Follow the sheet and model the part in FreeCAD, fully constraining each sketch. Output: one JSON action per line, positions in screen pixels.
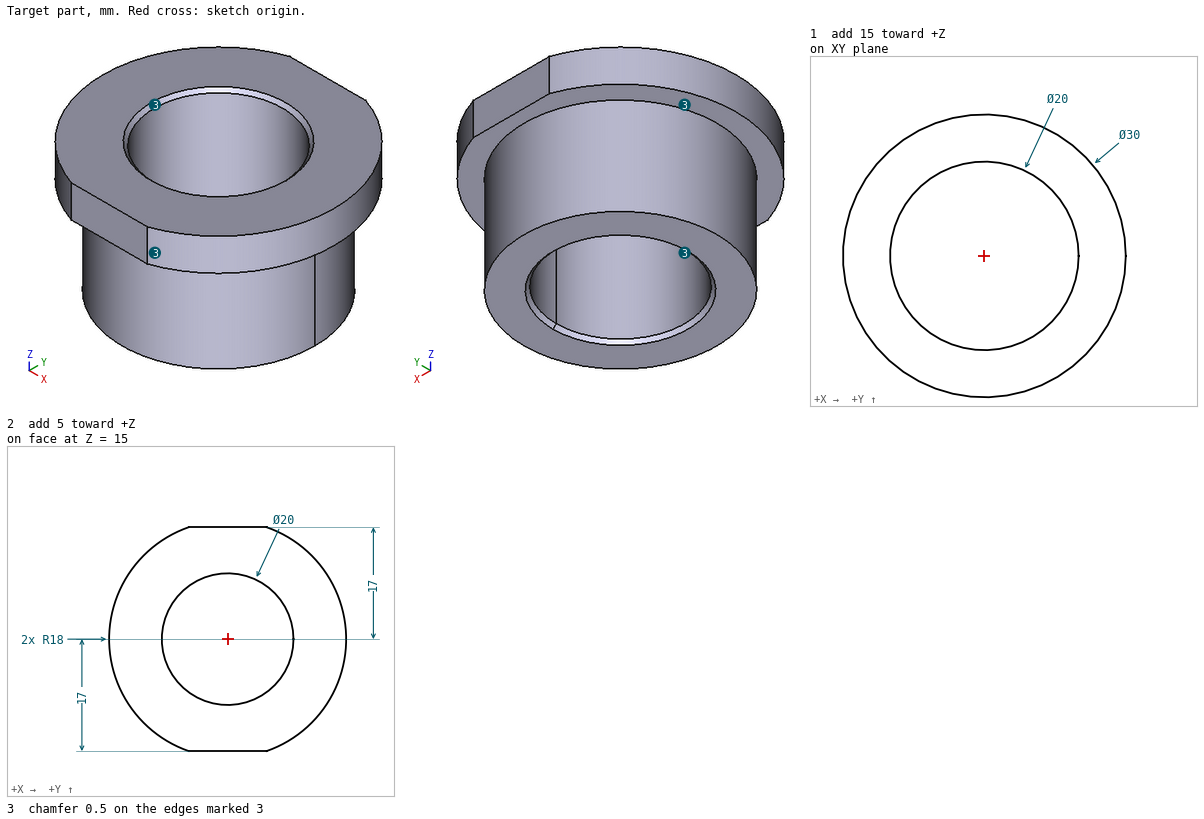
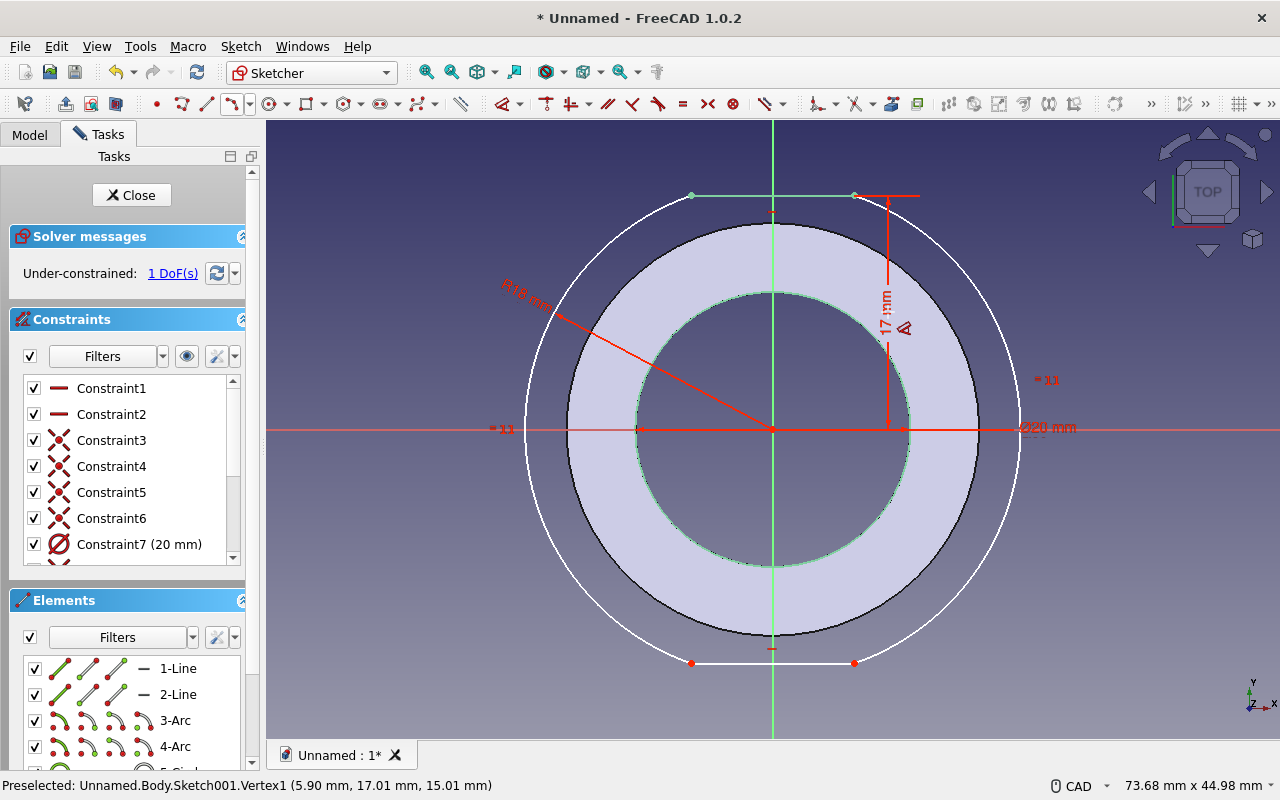
{"action": "left_click", "coordinate": [692, 664]}
{"action": "left_click", "coordinate": [658, 547]}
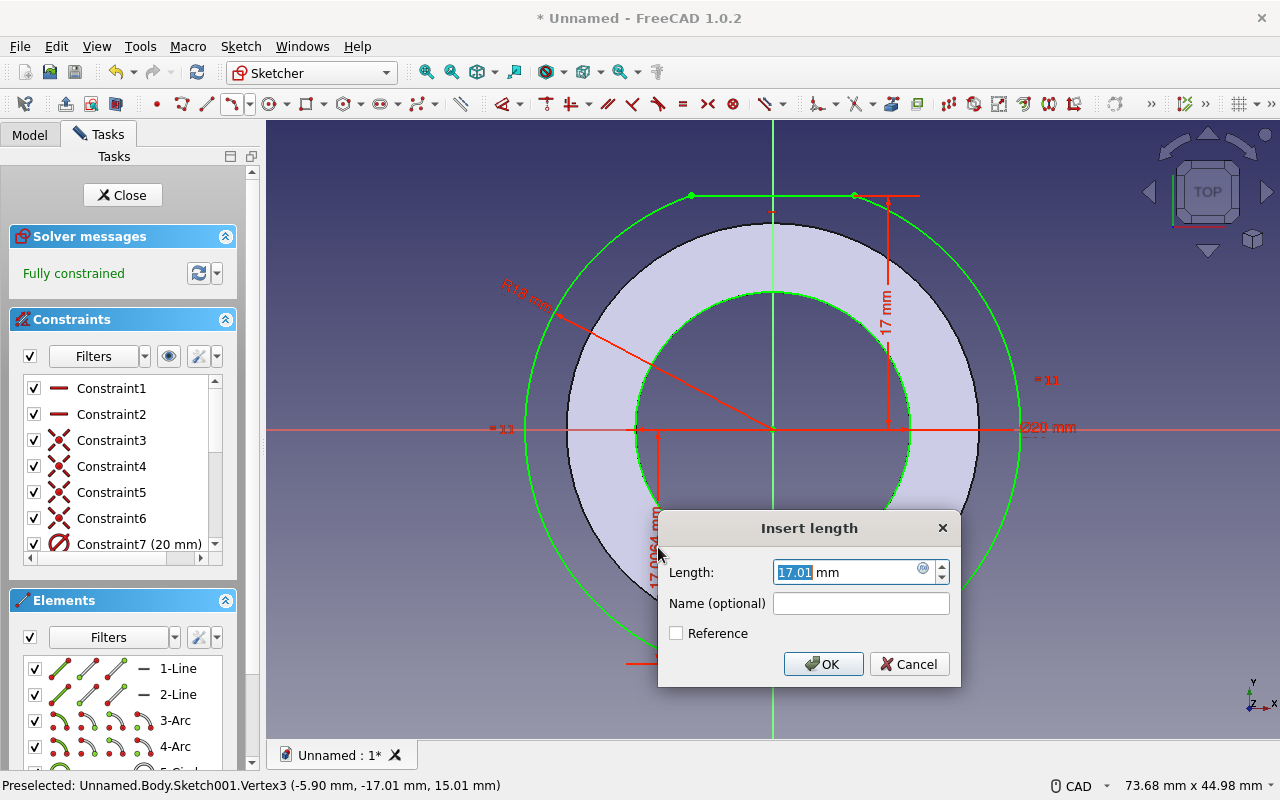
{"action": "type", "text": "17"}
{"action": "key", "text": "Return"}
{"action": "key", "text": "Escape"}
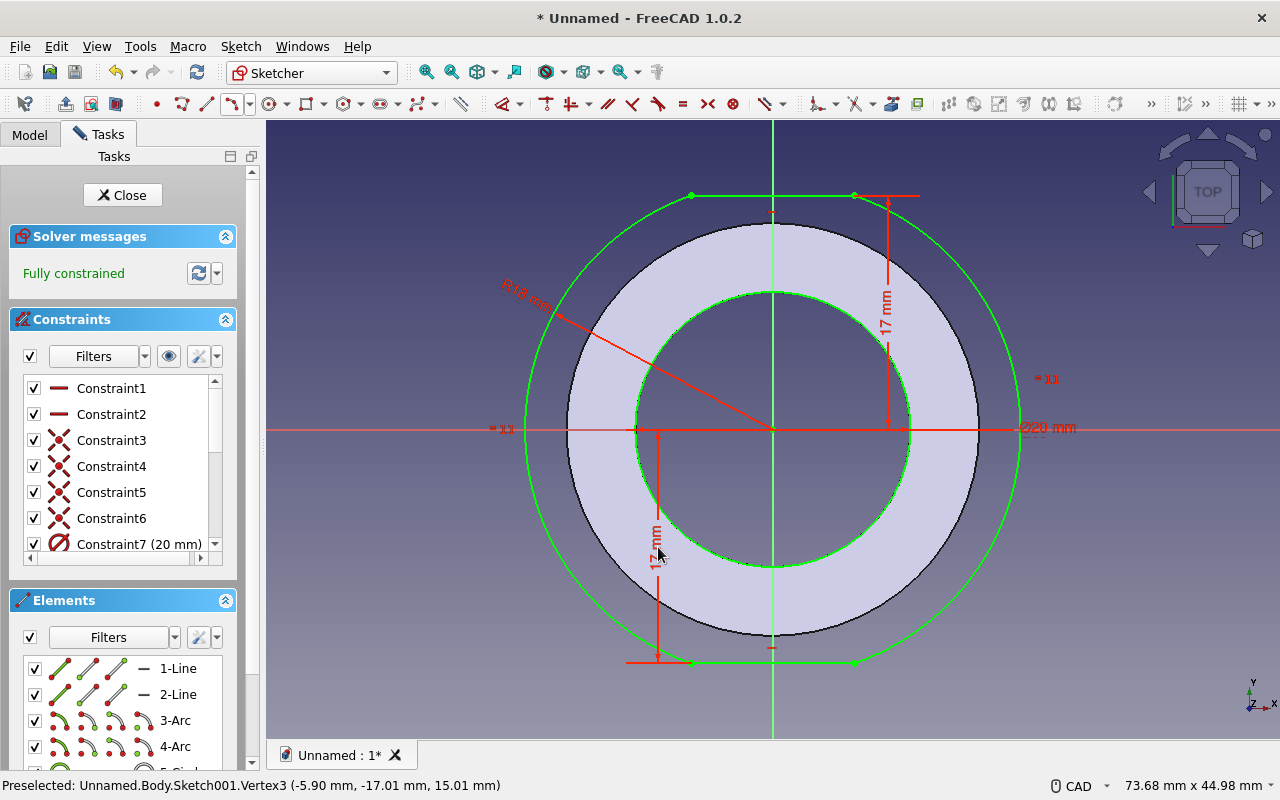
{"action": "left_click", "coordinate": [123, 195]}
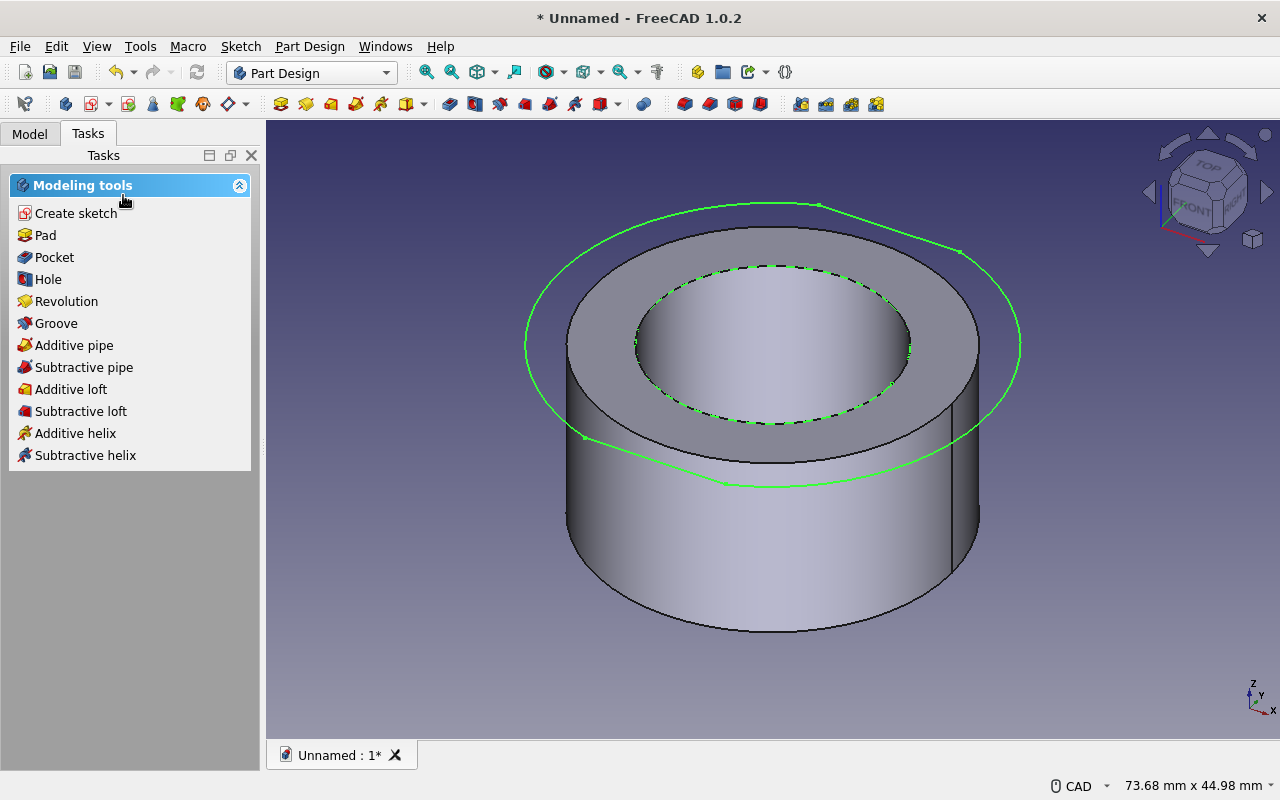
{"action": "left_click", "coordinate": [281, 104]}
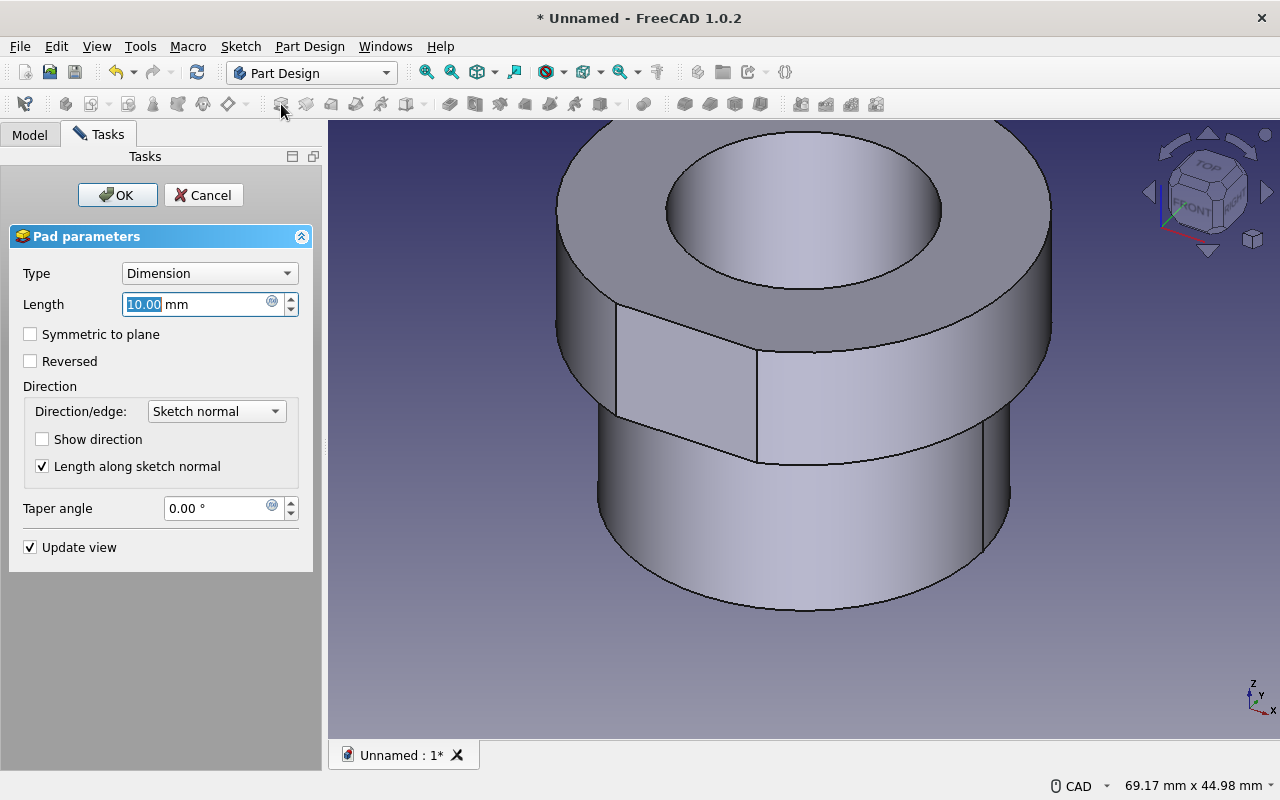
{"action": "type", "text": "5"}
{"action": "key", "text": "Tab"}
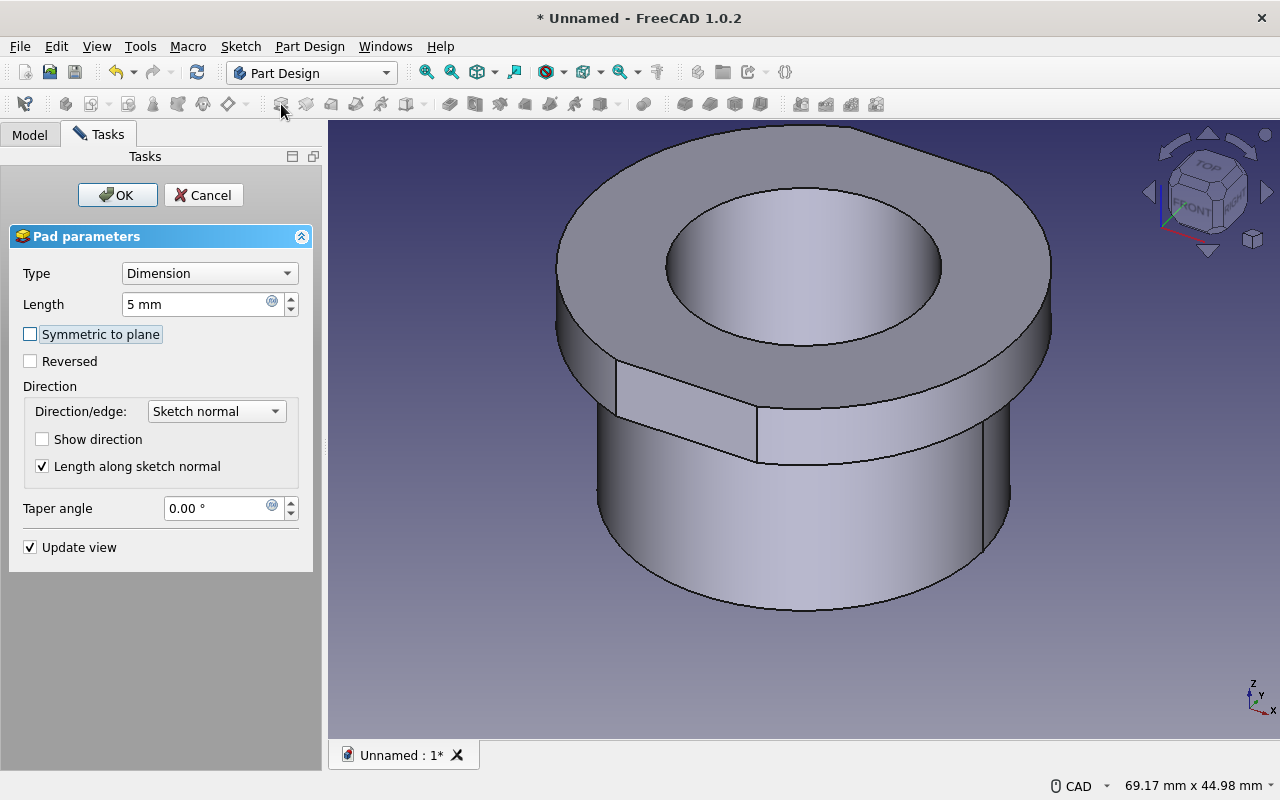
{"action": "left_click", "coordinate": [118, 195]}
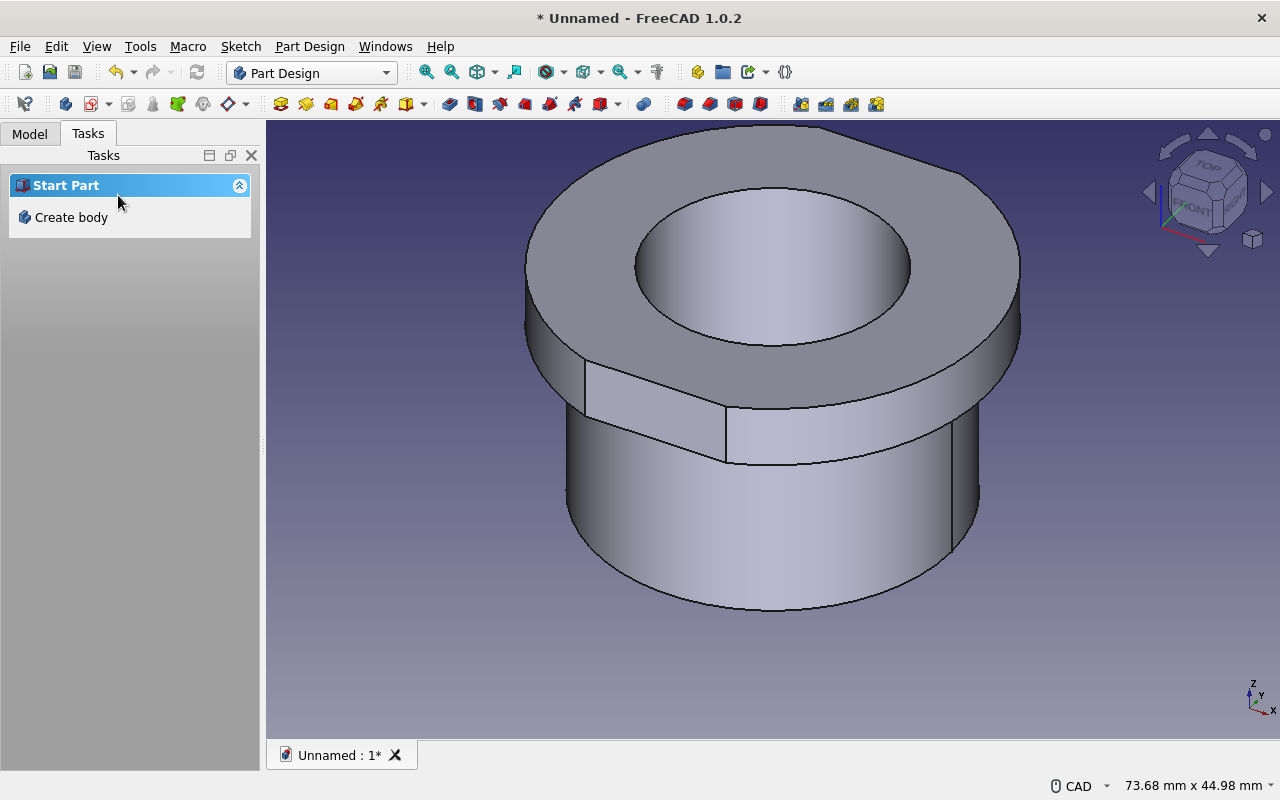
{"action": "left_click", "coordinate": [427, 72]}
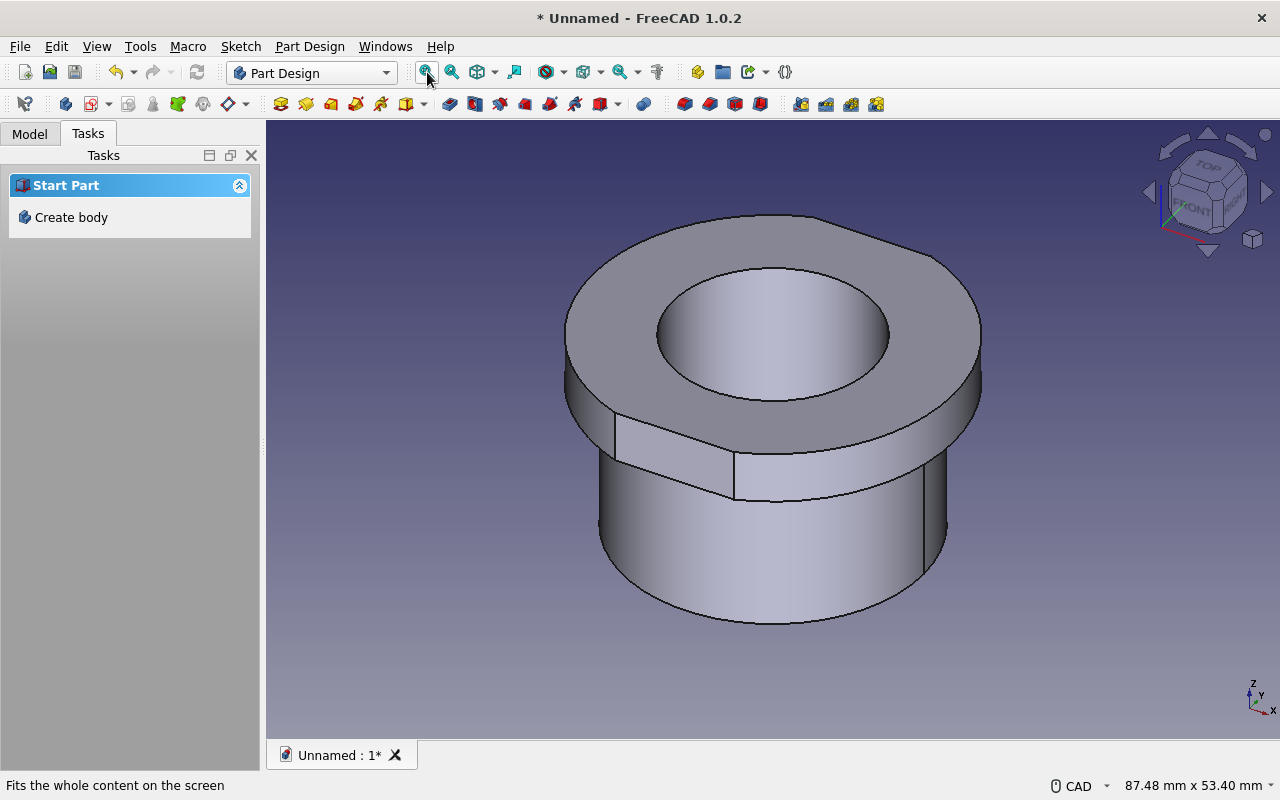
{"action": "left_click", "coordinate": [673, 300]}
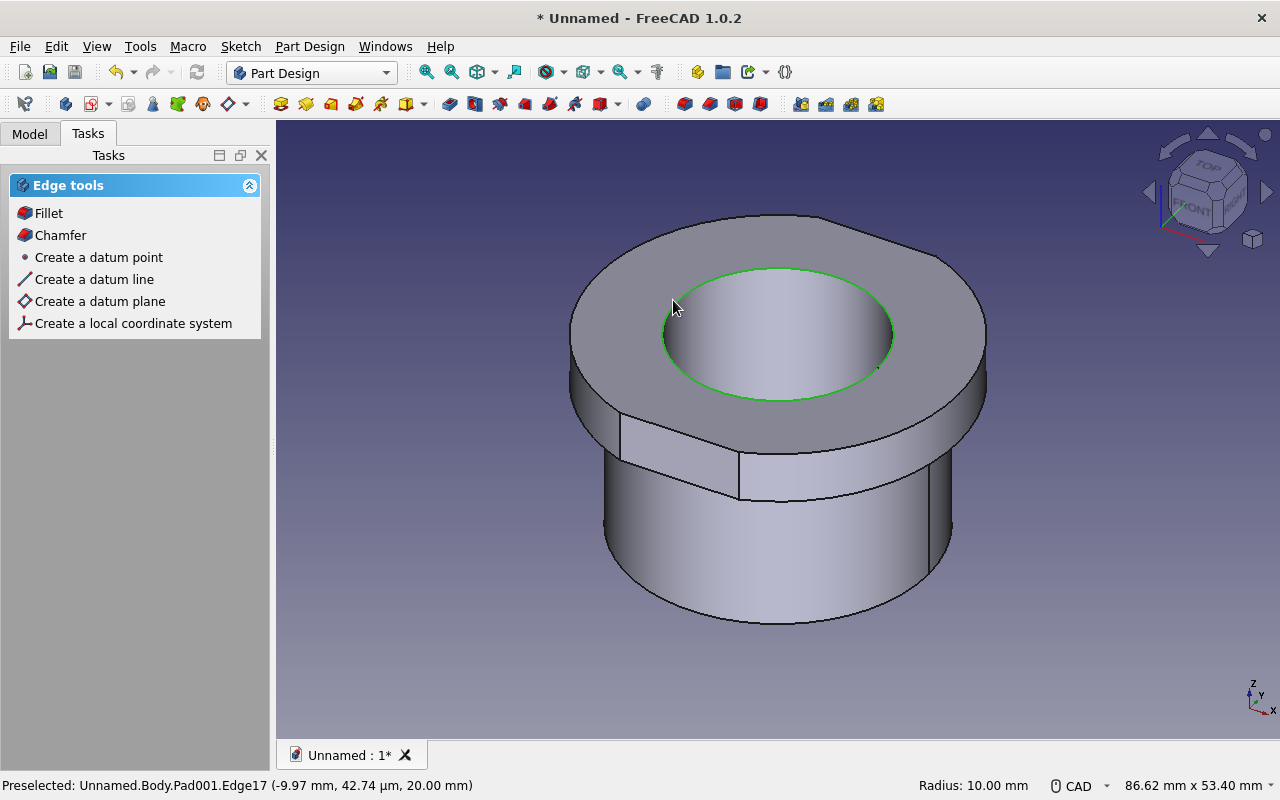
{"action": "key", "text": "0"}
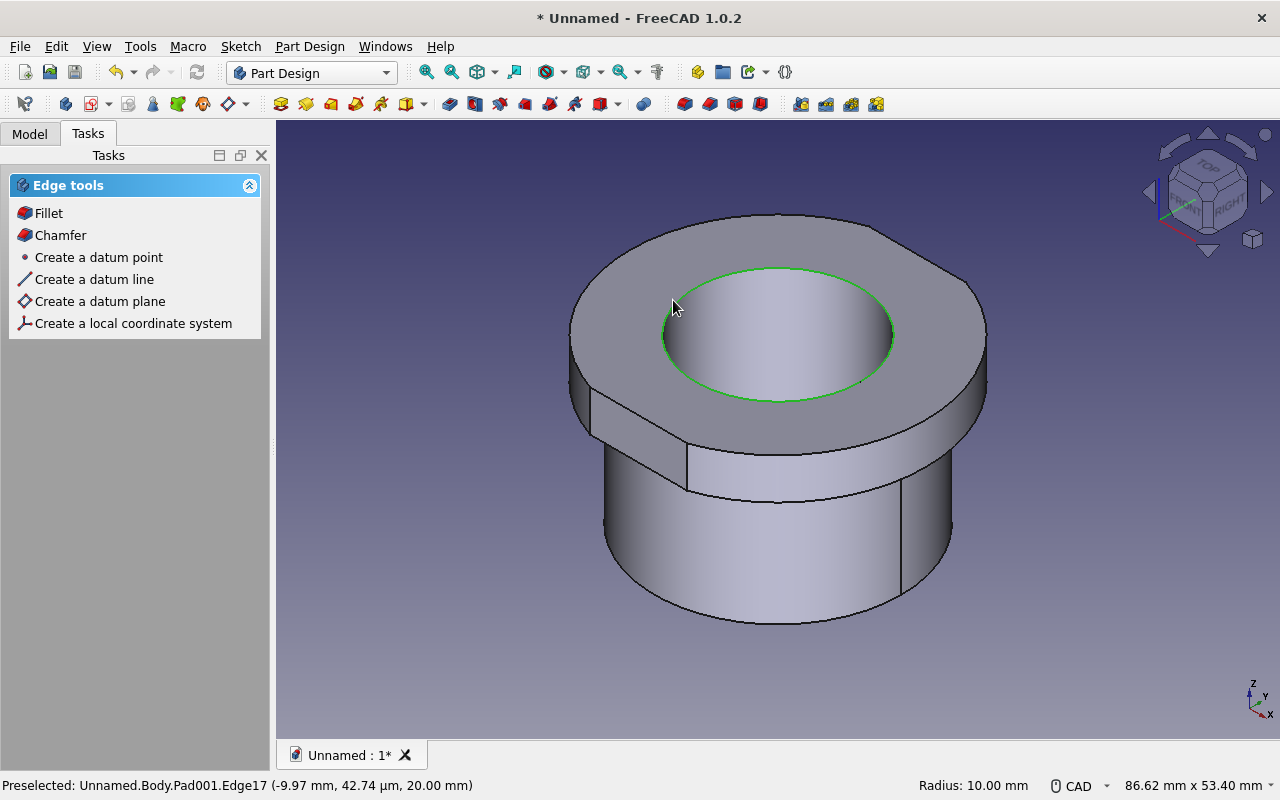
{"action": "key", "text": "2"}